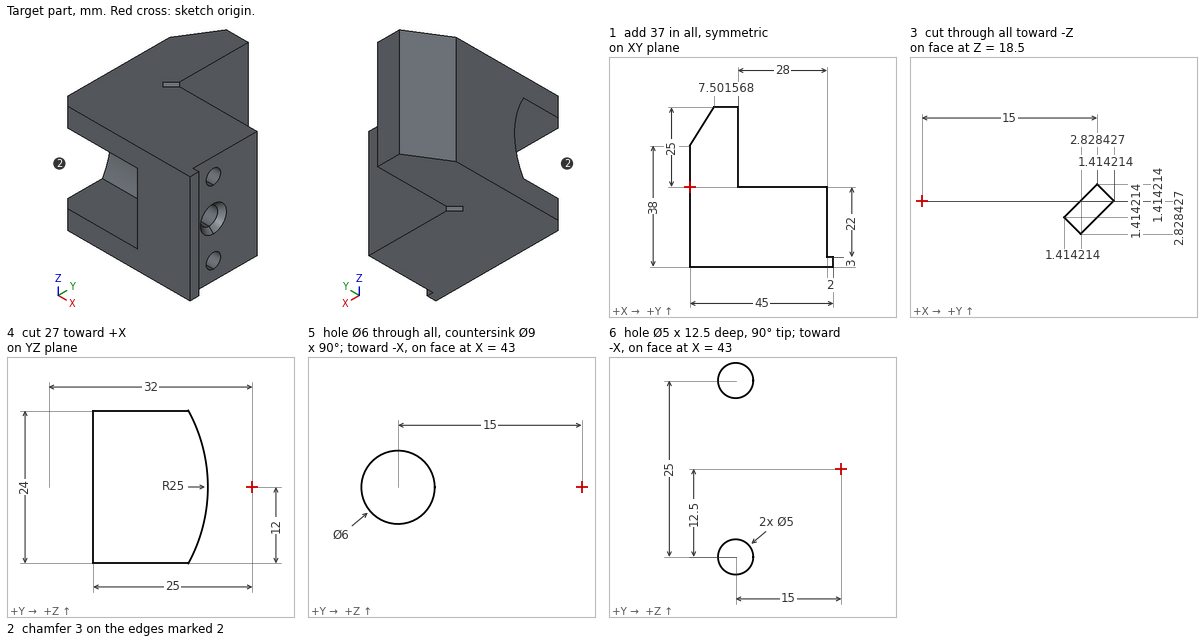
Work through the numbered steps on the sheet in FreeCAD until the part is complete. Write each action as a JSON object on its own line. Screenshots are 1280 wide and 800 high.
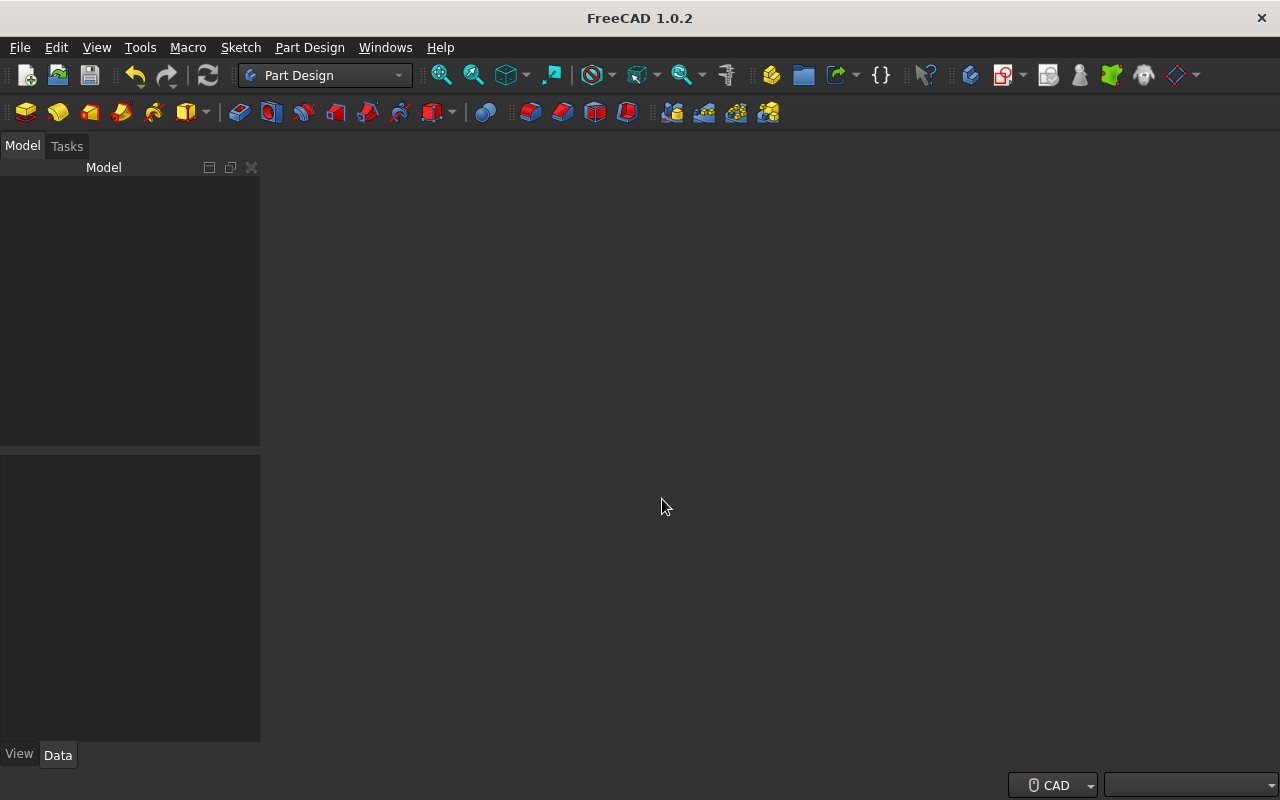
{"action": "left_click", "coordinate": [26, 76]}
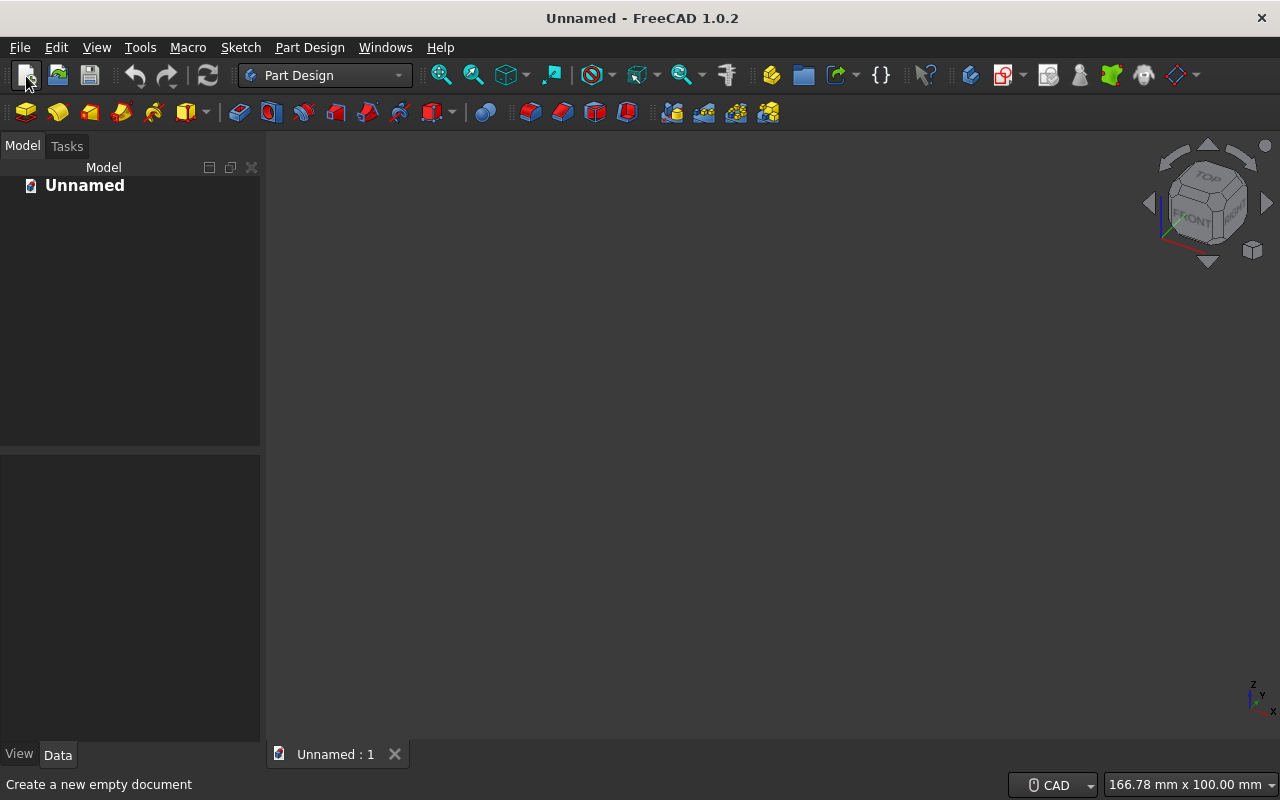
{"action": "left_click", "coordinate": [1004, 76]}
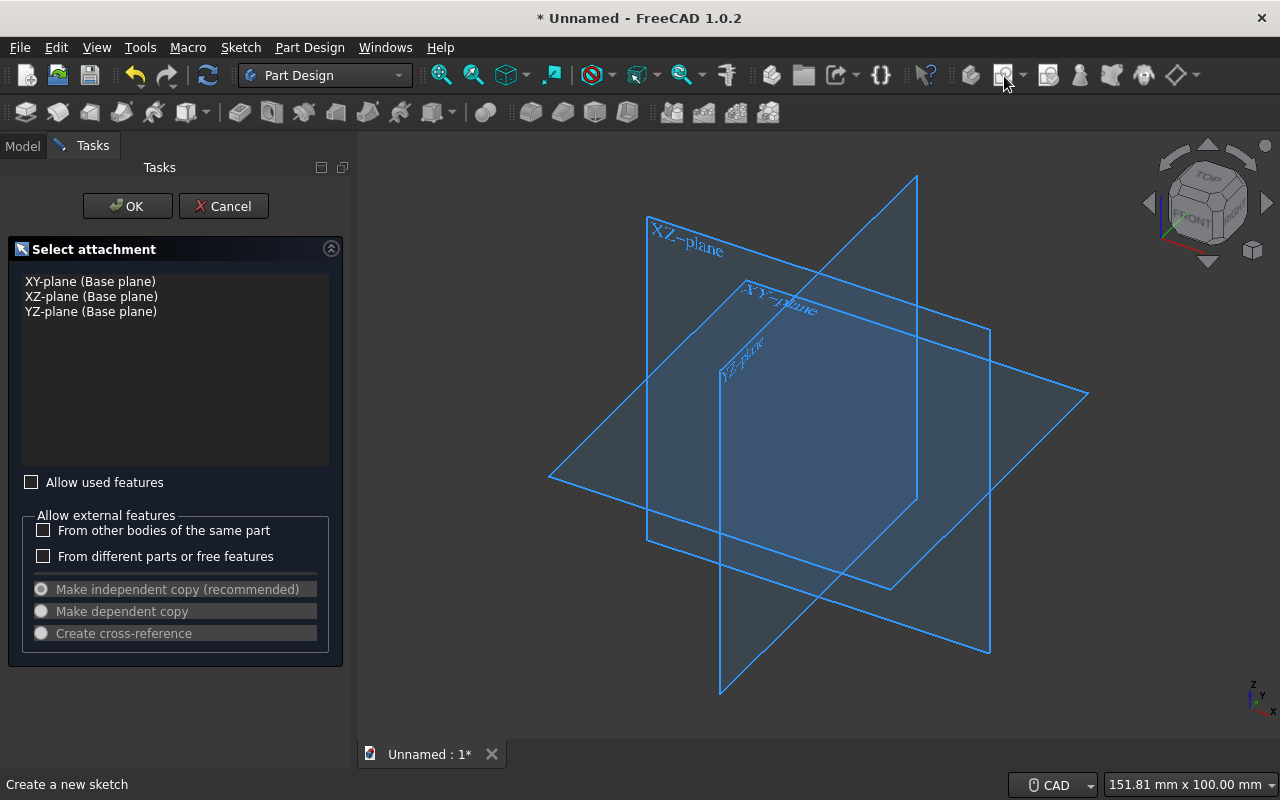
{"action": "left_click", "coordinate": [82, 282]}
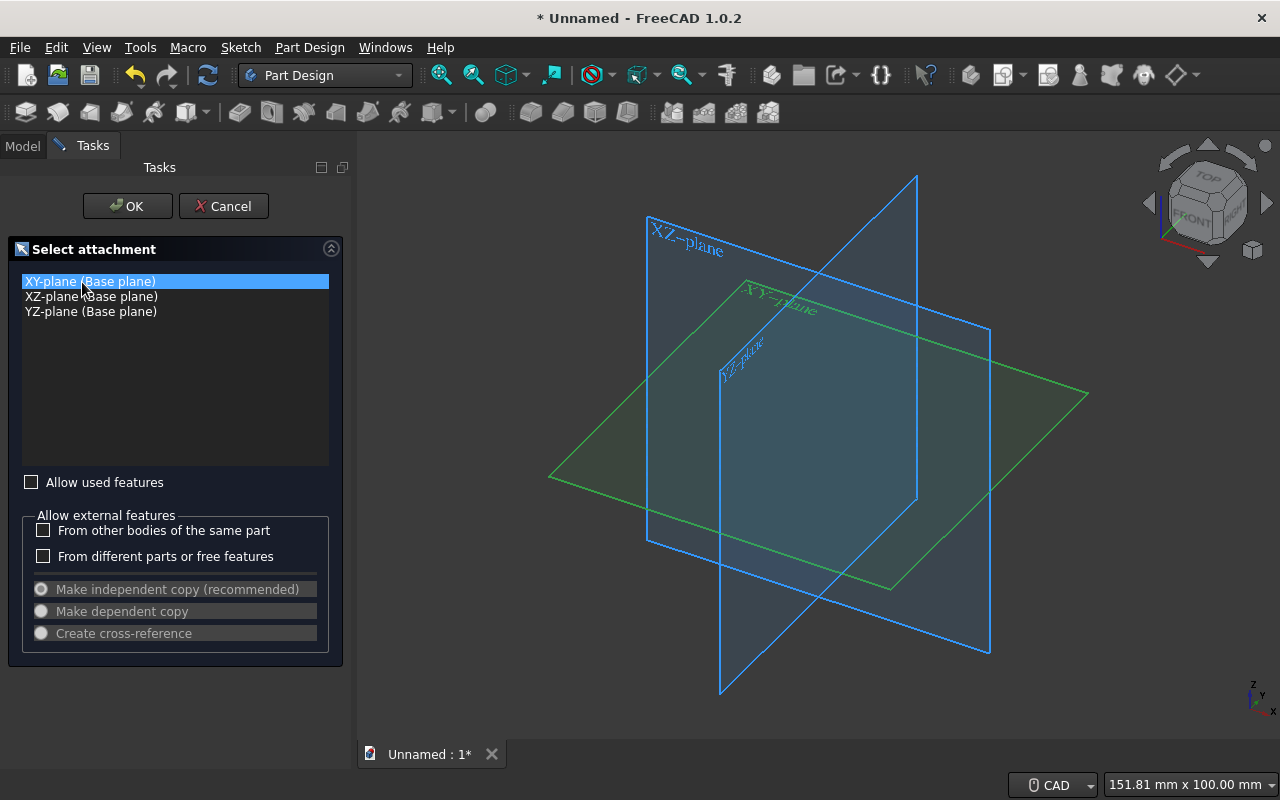
{"action": "left_click", "coordinate": [128, 206]}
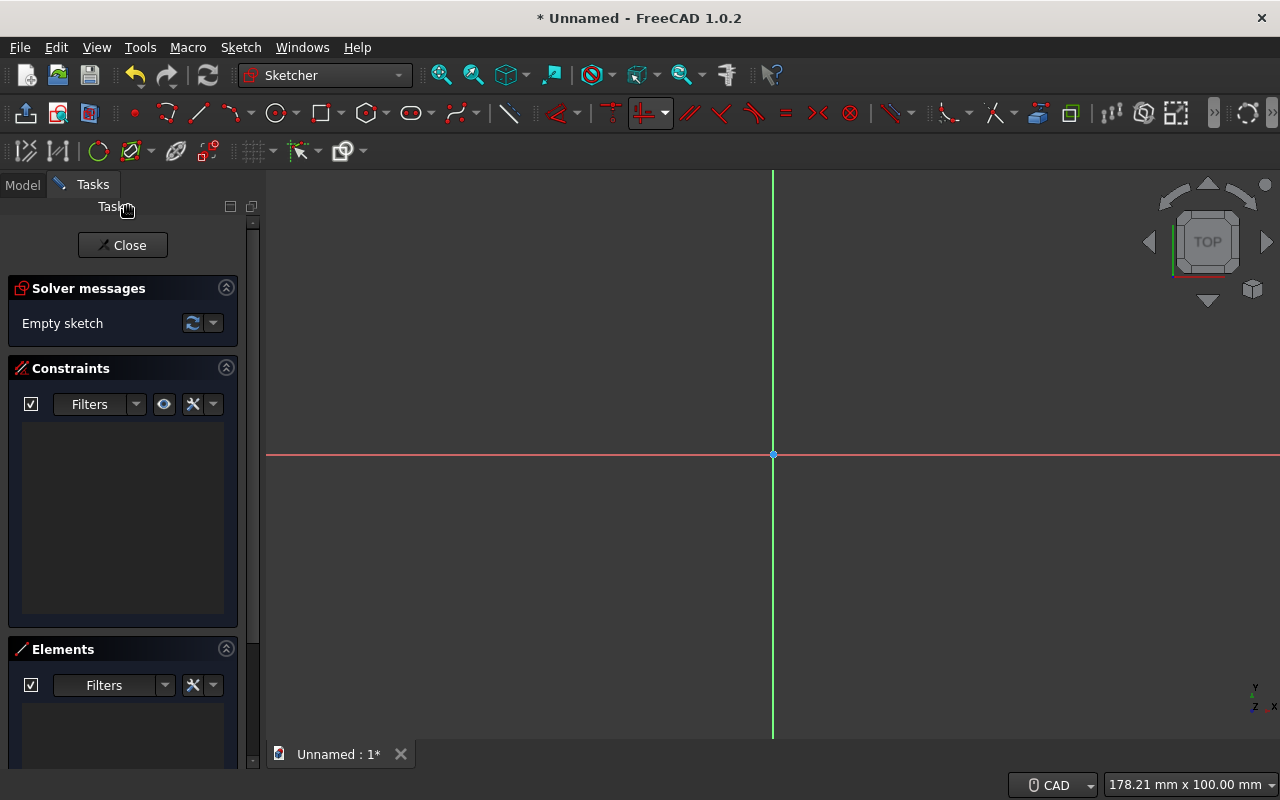
{"action": "left_click", "coordinate": [168, 114]}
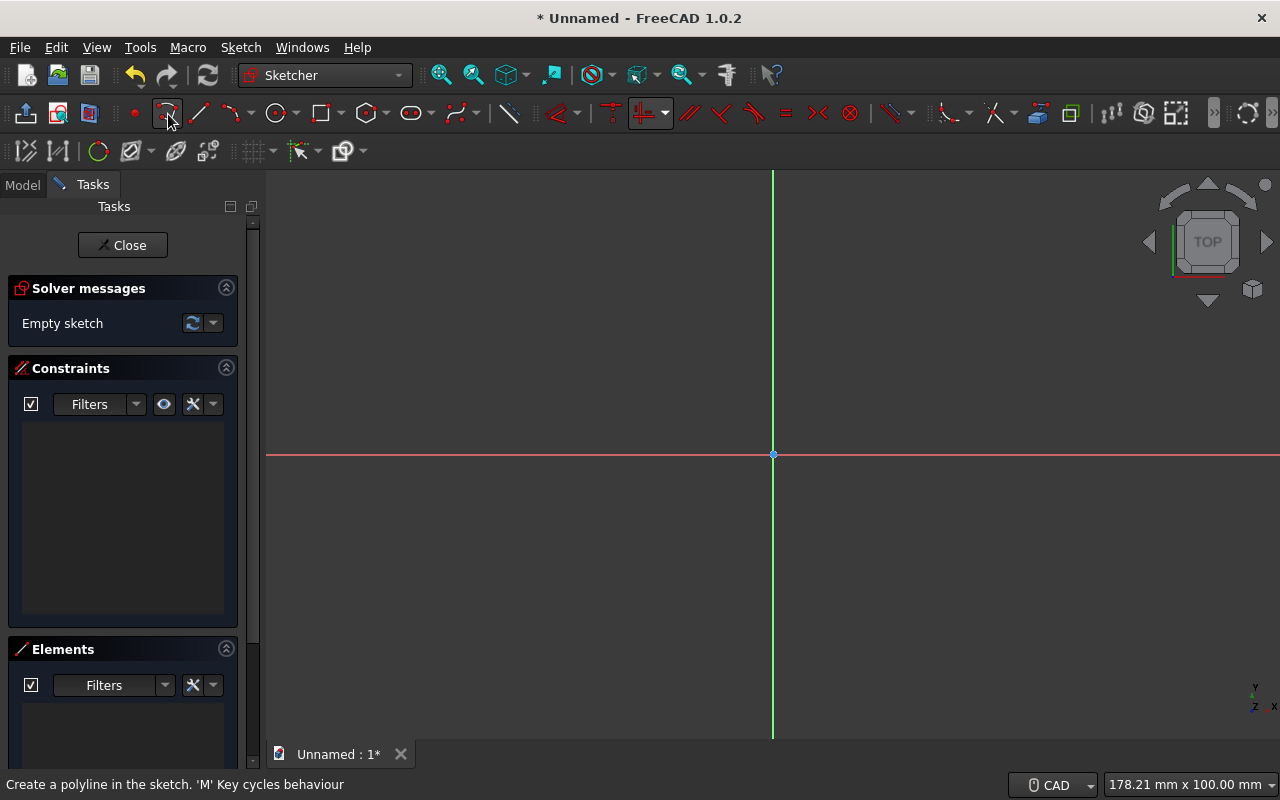
{"action": "left_click", "coordinate": [773, 381]}
{"action": "left_click", "coordinate": [782, 597]}
{"action": "left_click", "coordinate": [1029, 597]}
{"action": "left_click", "coordinate": [1029, 580]}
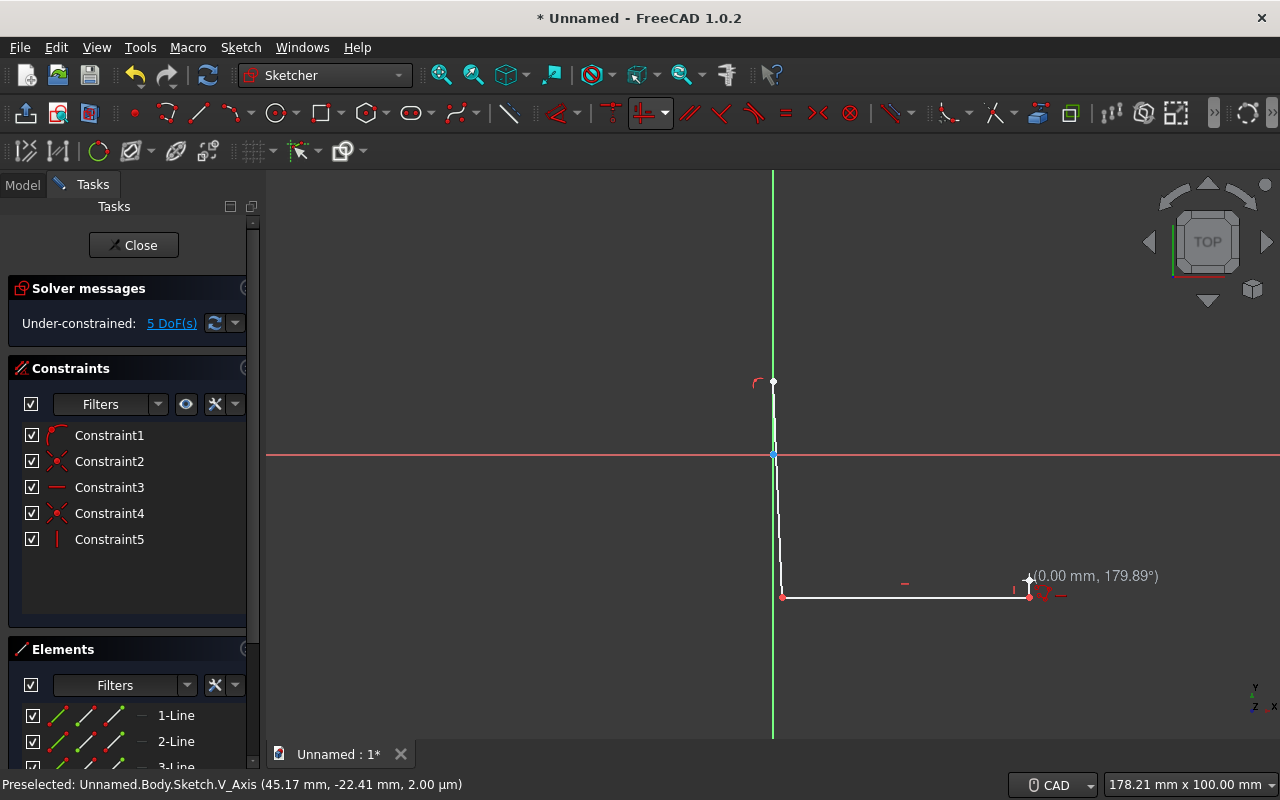
{"action": "scroll", "coordinate": [1018, 580], "scroll_direction": "up", "scroll_amount": 2}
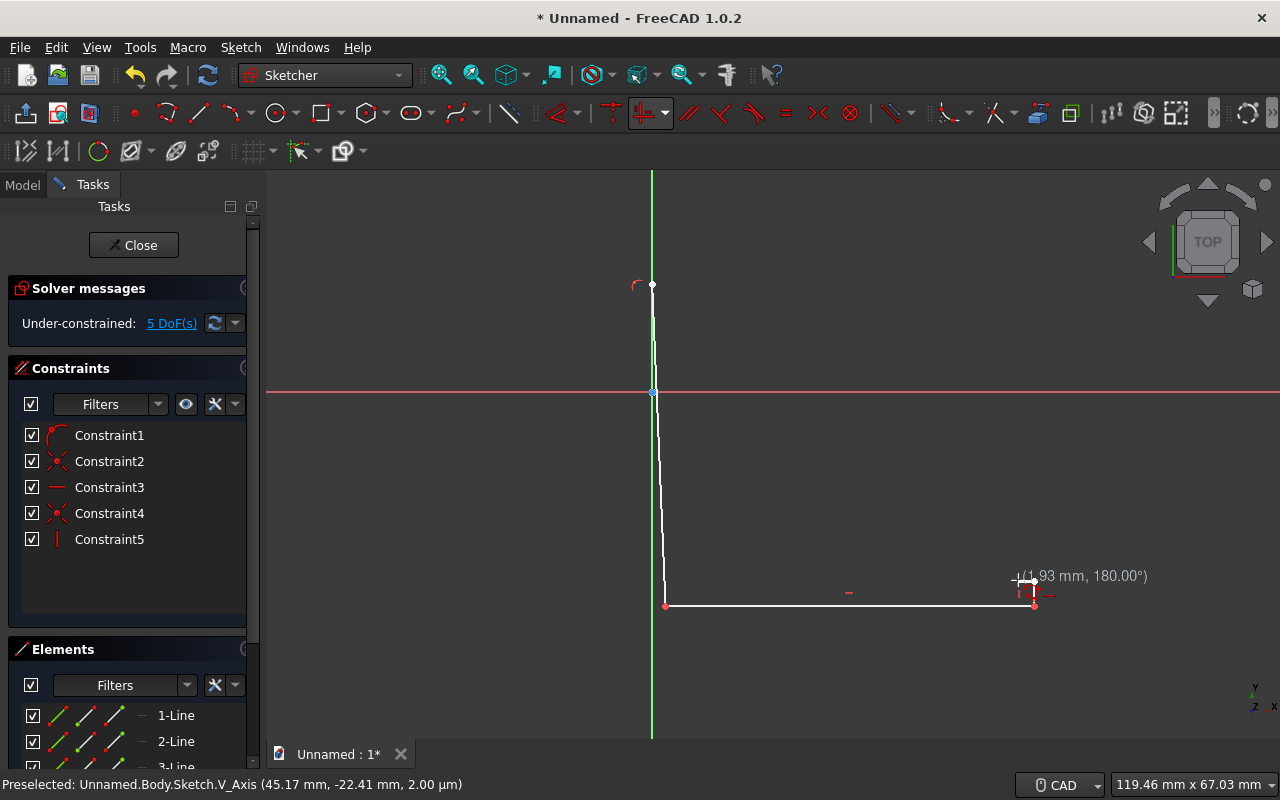
{"action": "left_click", "coordinate": [1017, 580]}
{"action": "left_click", "coordinate": [1017, 392]}
{"action": "left_click", "coordinate": [779, 383]}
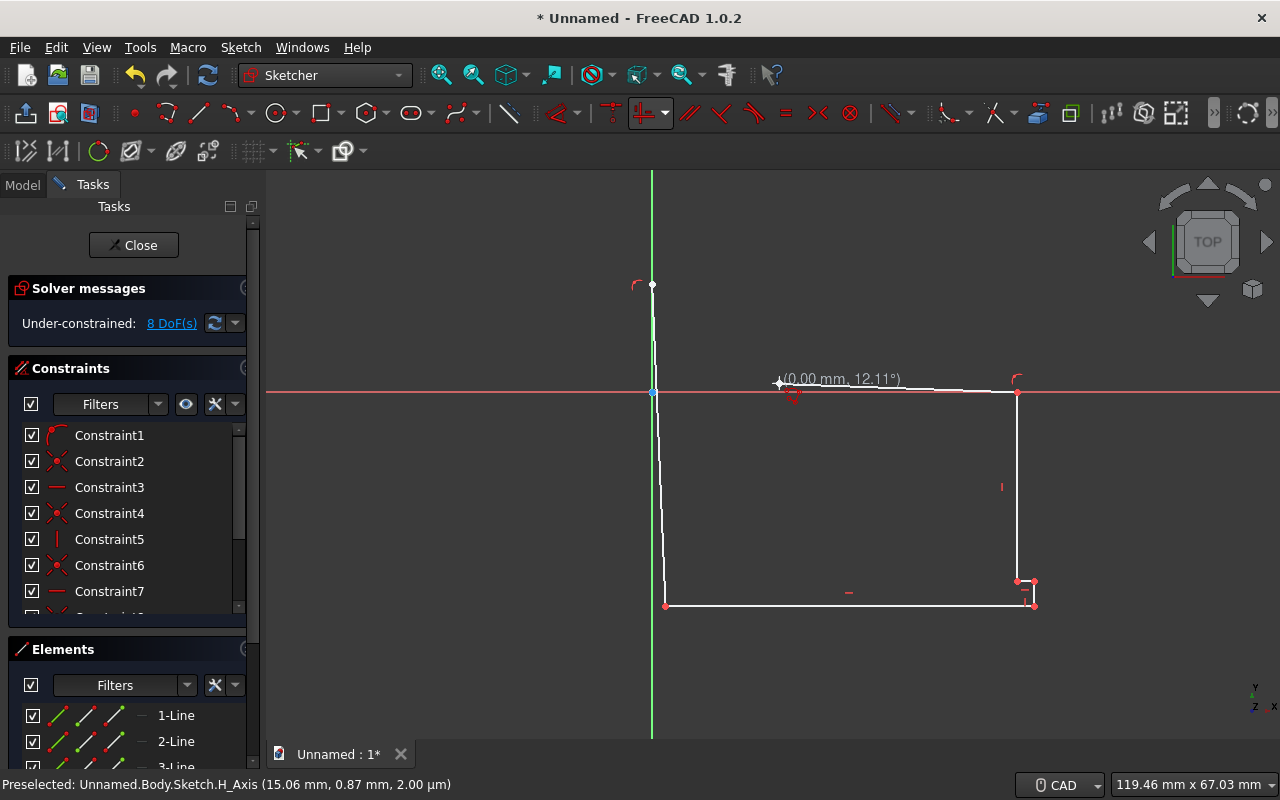
{"action": "scroll", "coordinate": [294, 711], "scroll_direction": "down", "scroll_amount": 1}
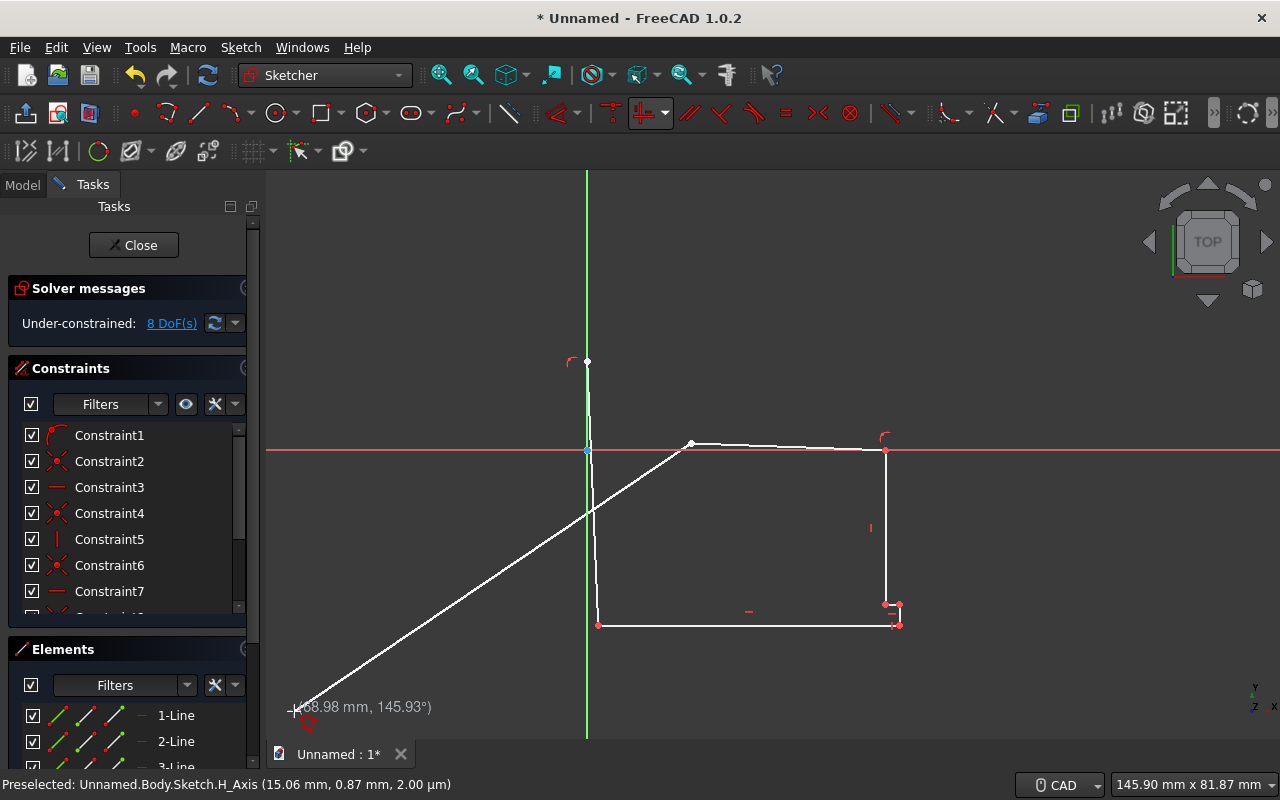
{"action": "left_click", "coordinate": [691, 277]}
{"action": "left_click", "coordinate": [639, 277]}
{"action": "left_click", "coordinate": [587, 362]}
{"action": "key", "text": "Escape"}
{"action": "key", "text": "Escape"}